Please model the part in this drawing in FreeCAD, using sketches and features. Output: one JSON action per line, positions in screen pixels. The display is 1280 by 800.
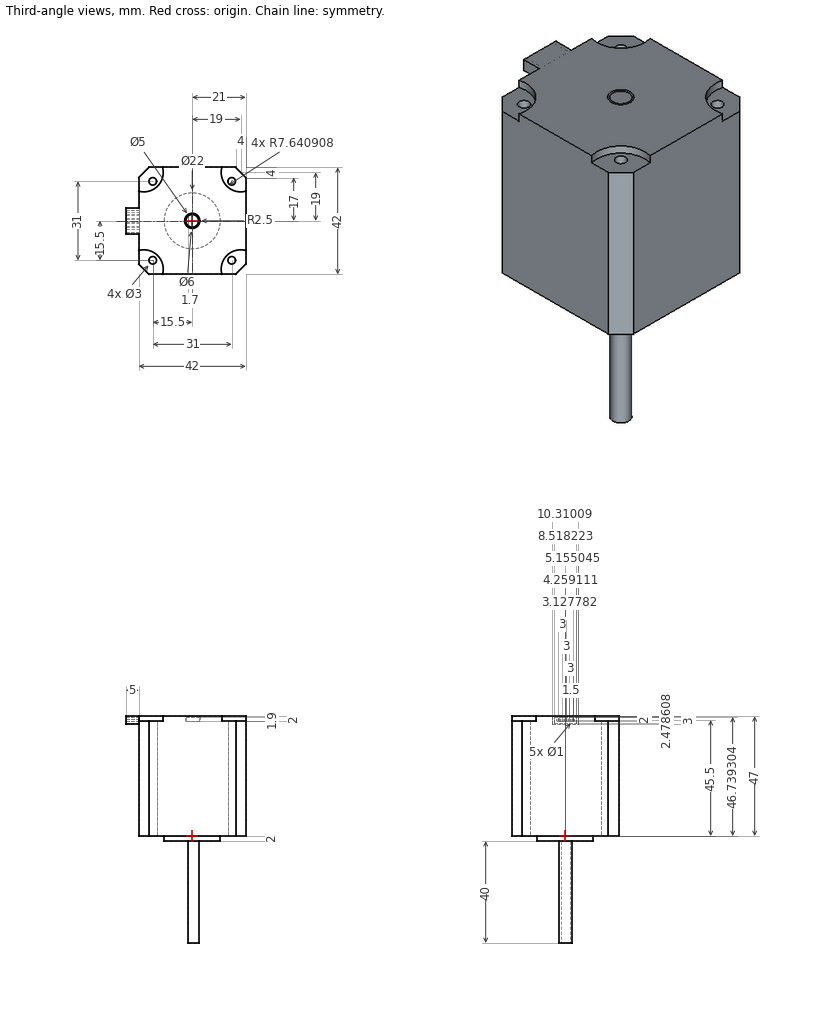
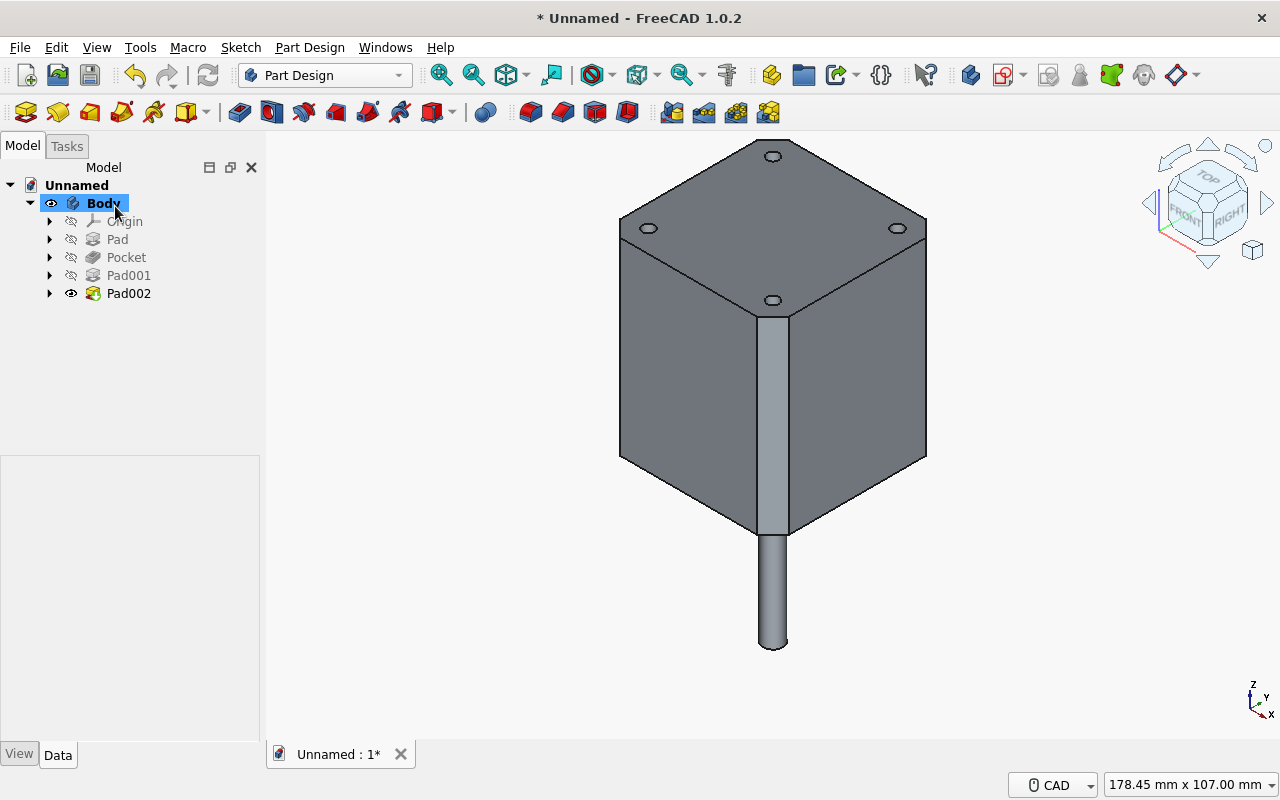
{"action": "left_click", "coordinate": [773, 228]}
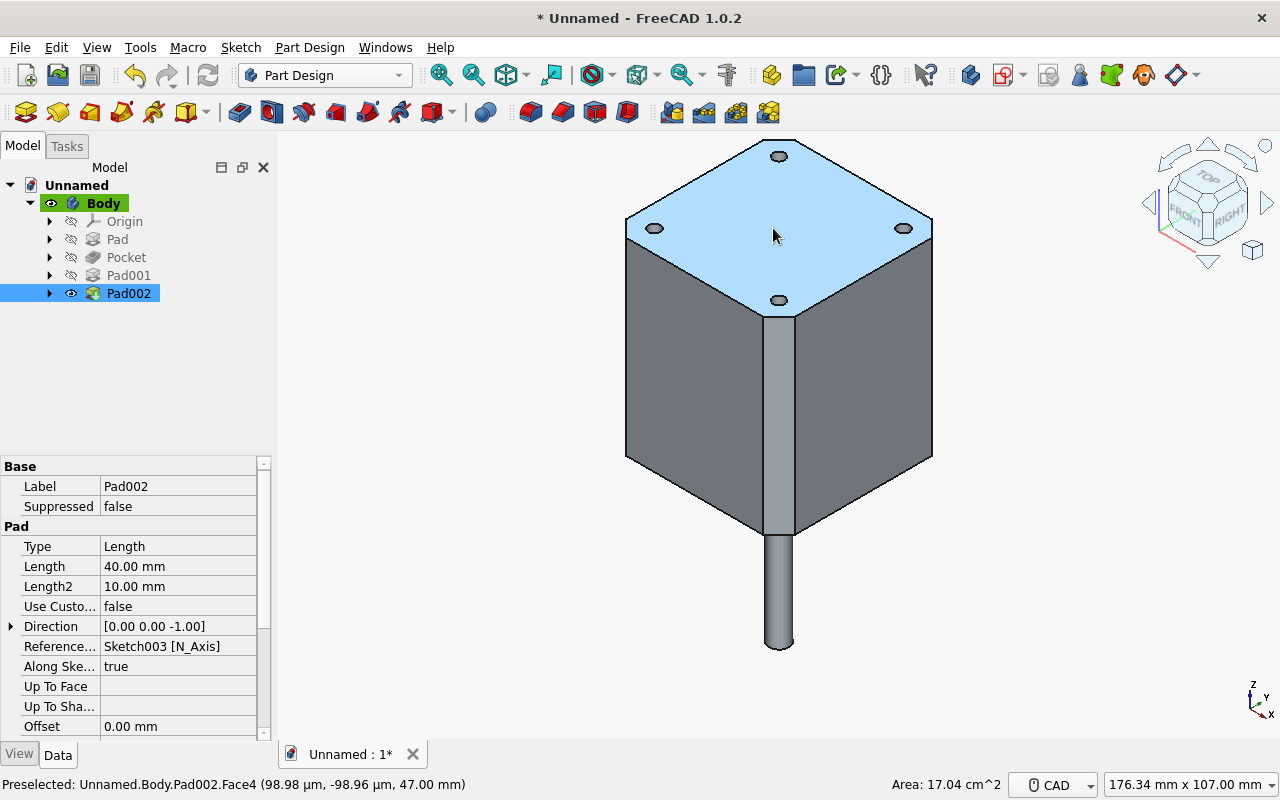
{"action": "left_click", "coordinate": [1004, 76]}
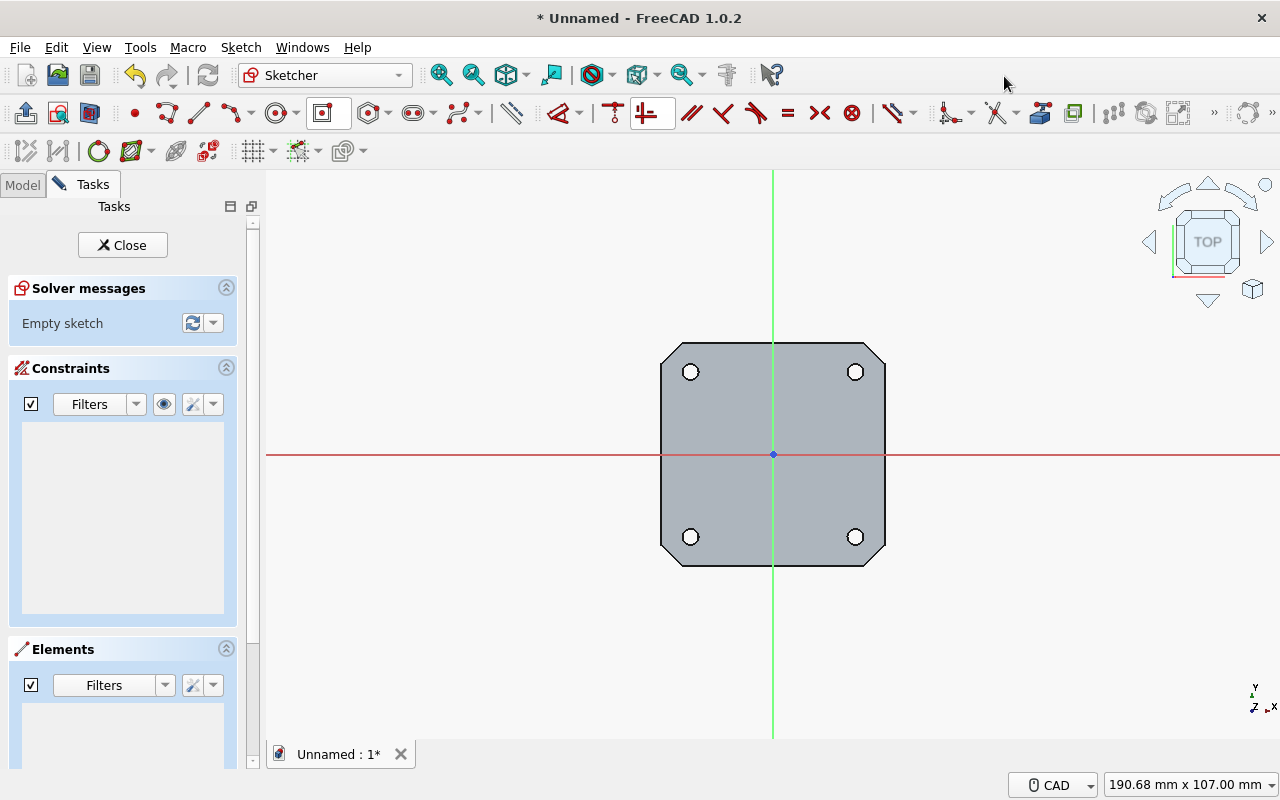
{"action": "scroll", "coordinate": [912, 455], "scroll_direction": "up", "scroll_amount": 2}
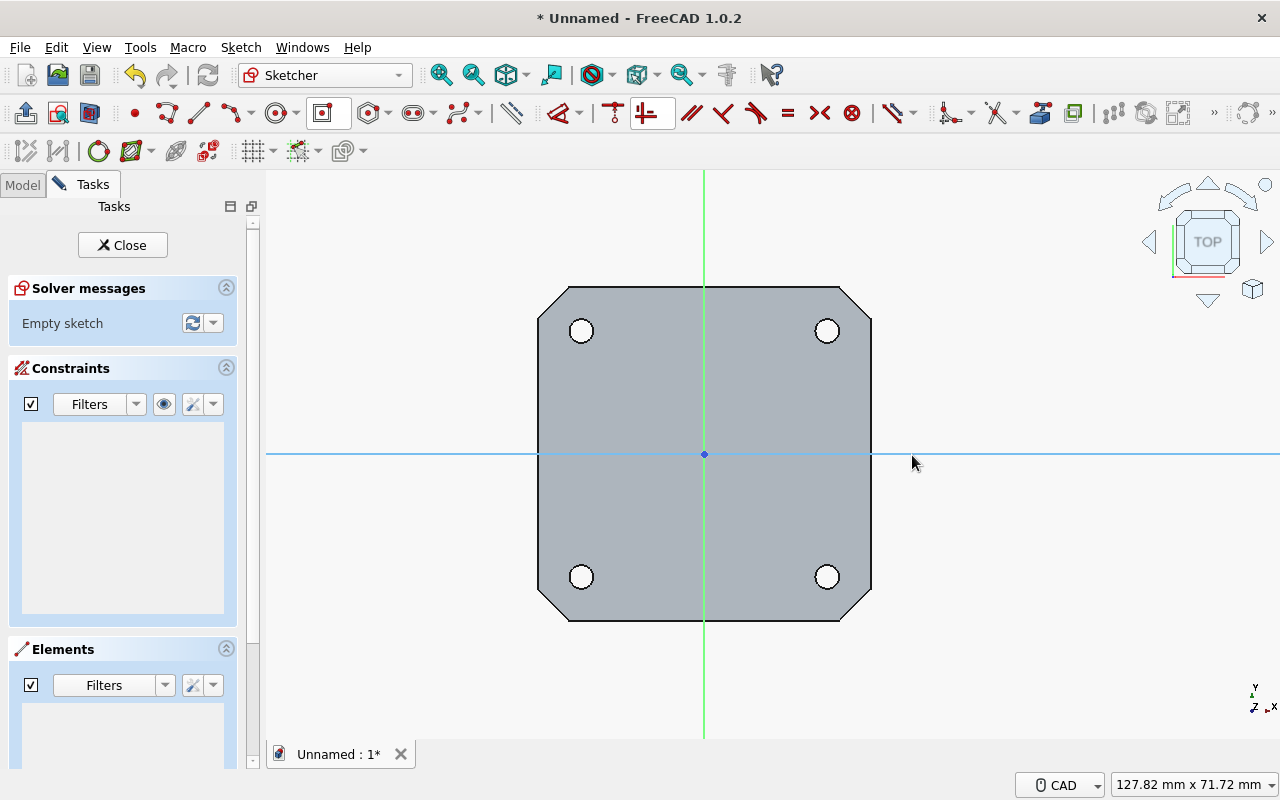
{"action": "left_click", "coordinate": [168, 114]}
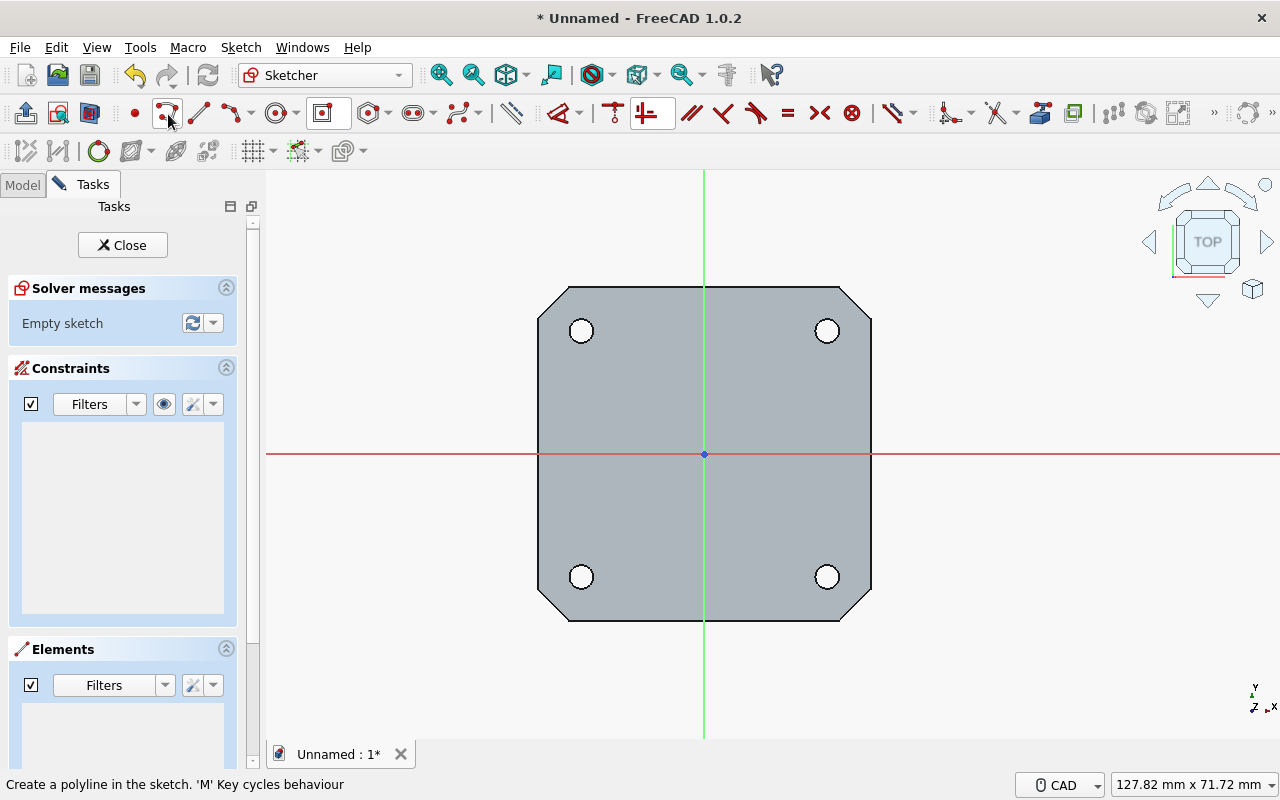
{"action": "left_click", "coordinate": [871, 362]}
{"action": "left_click", "coordinate": [871, 319]}
{"action": "left_click", "coordinate": [839, 287]}
{"action": "left_click", "coordinate": [797, 287]}
{"action": "right_click", "coordinate": [797, 287]}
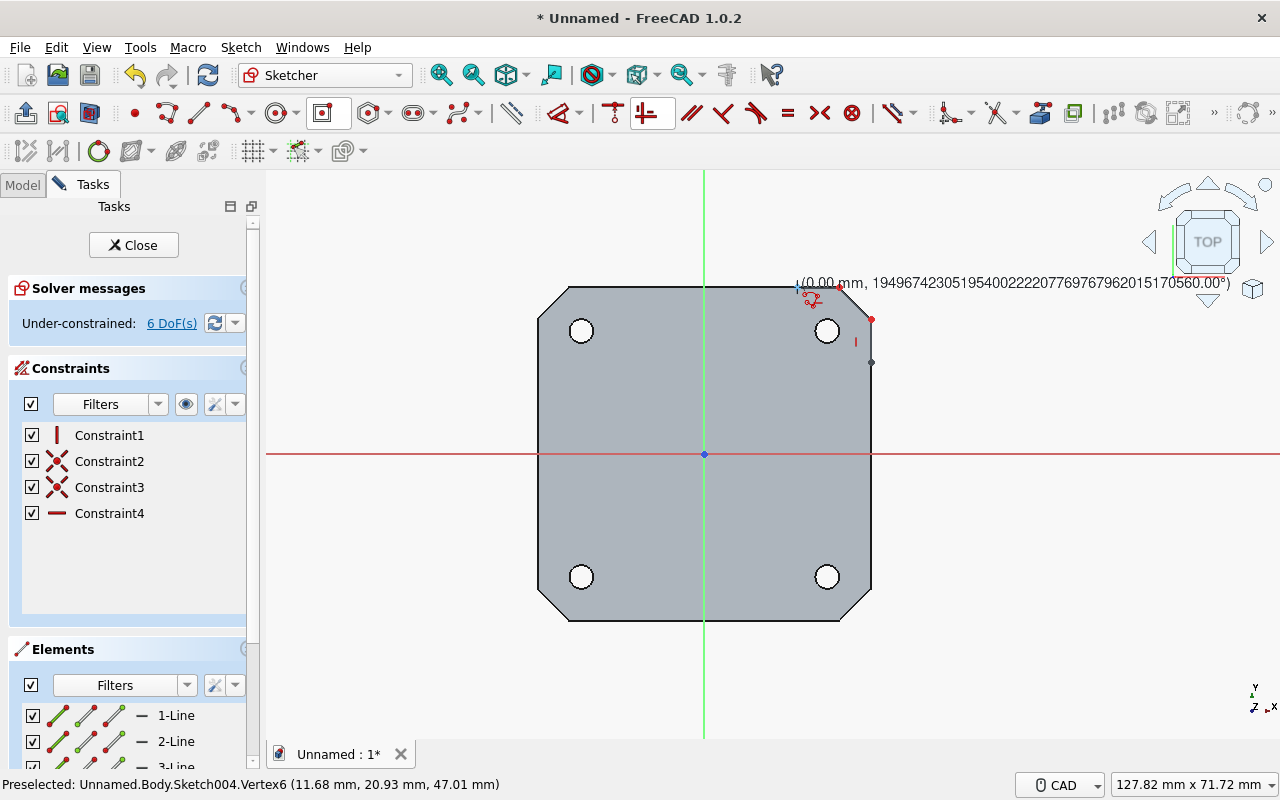
{"action": "left_click", "coordinate": [232, 114]}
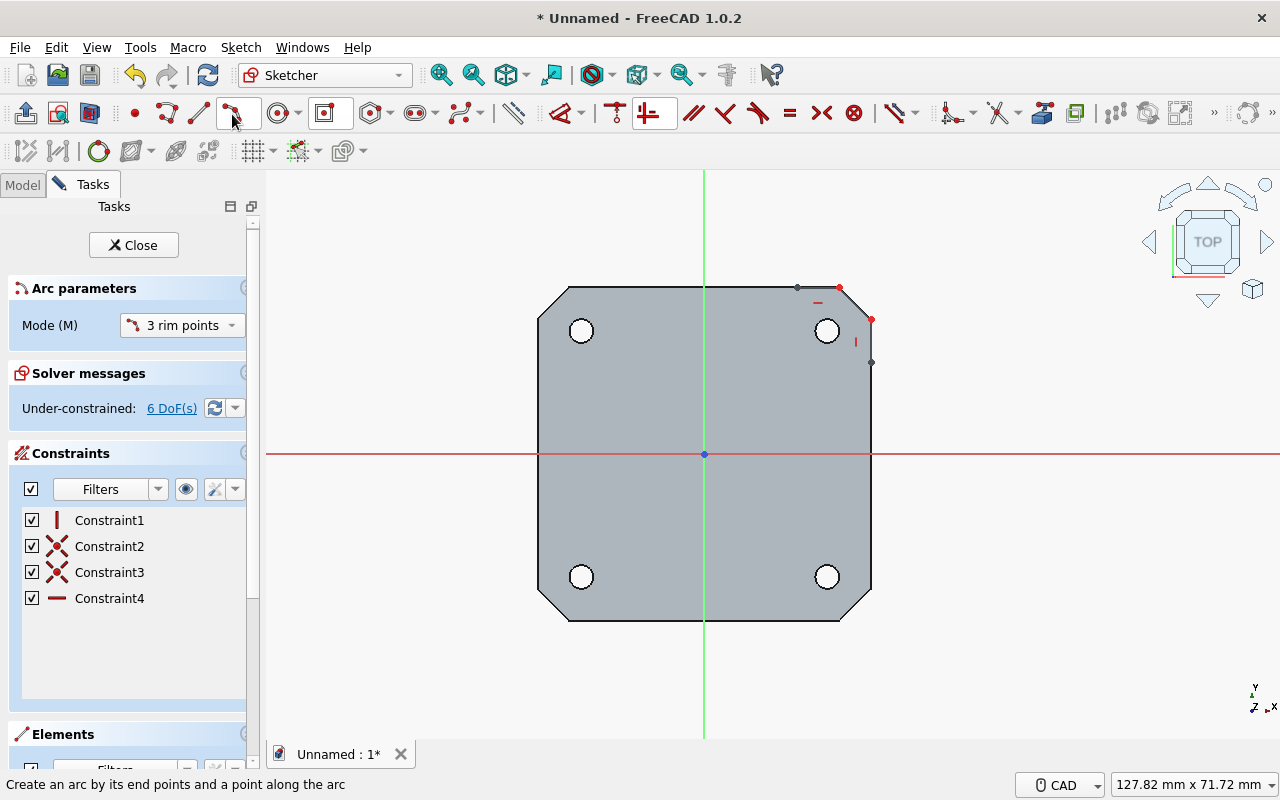
{"action": "left_click", "coordinate": [797, 288]}
{"action": "left_click", "coordinate": [871, 363]}
{"action": "left_click", "coordinate": [812, 346]}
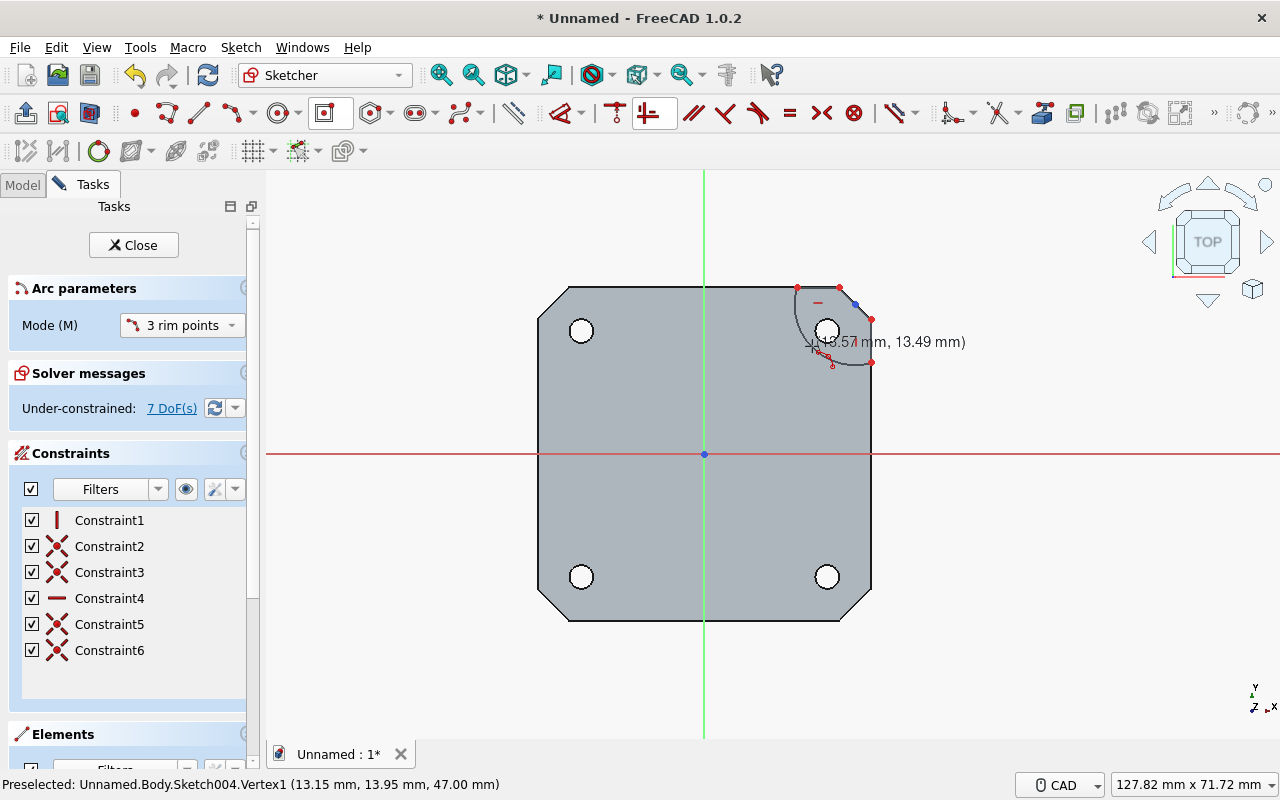
{"action": "left_click", "coordinate": [168, 114]}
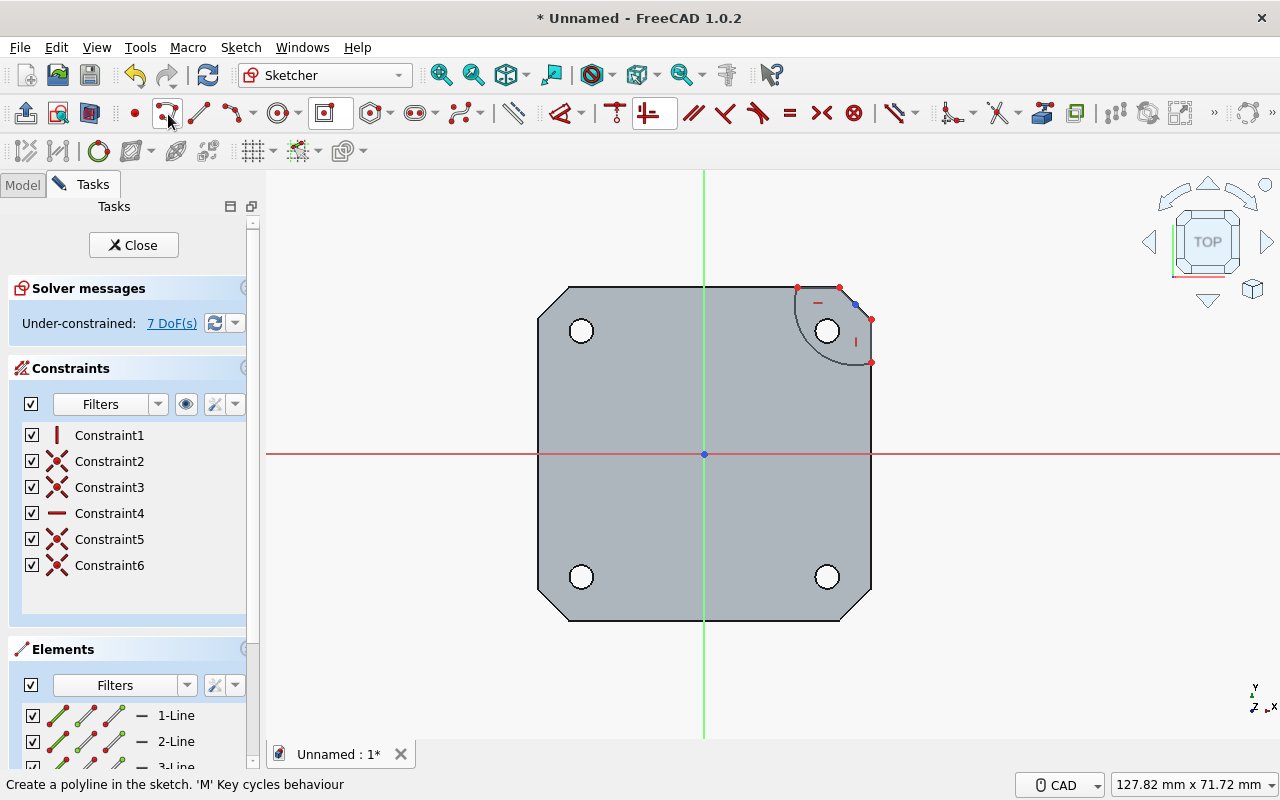
{"action": "left_click", "coordinate": [538, 546]}
{"action": "left_click", "coordinate": [538, 589]}
{"action": "left_click", "coordinate": [569, 621]}
{"action": "left_click", "coordinate": [612, 621]}
{"action": "right_click", "coordinate": [612, 621]}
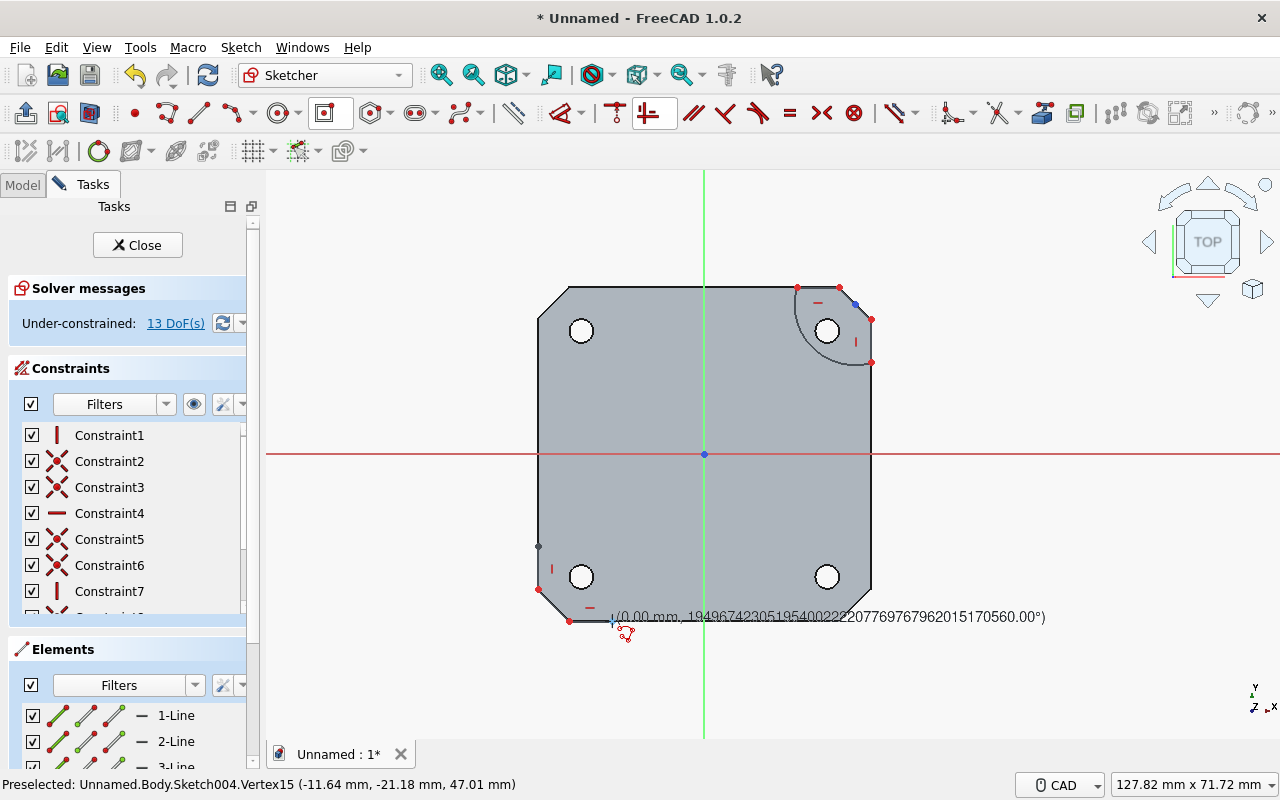
{"action": "left_click", "coordinate": [232, 114]}